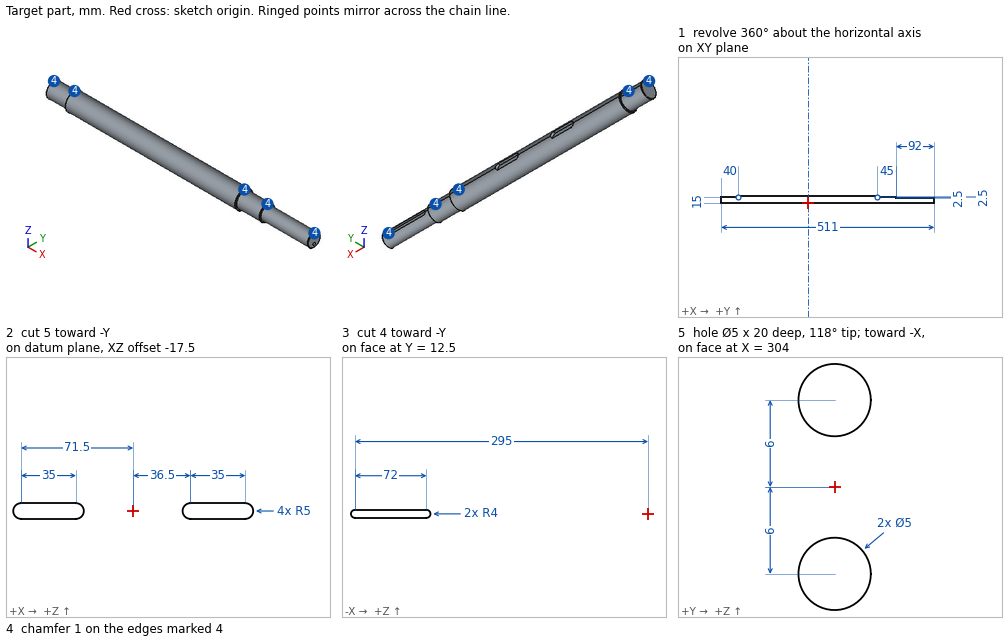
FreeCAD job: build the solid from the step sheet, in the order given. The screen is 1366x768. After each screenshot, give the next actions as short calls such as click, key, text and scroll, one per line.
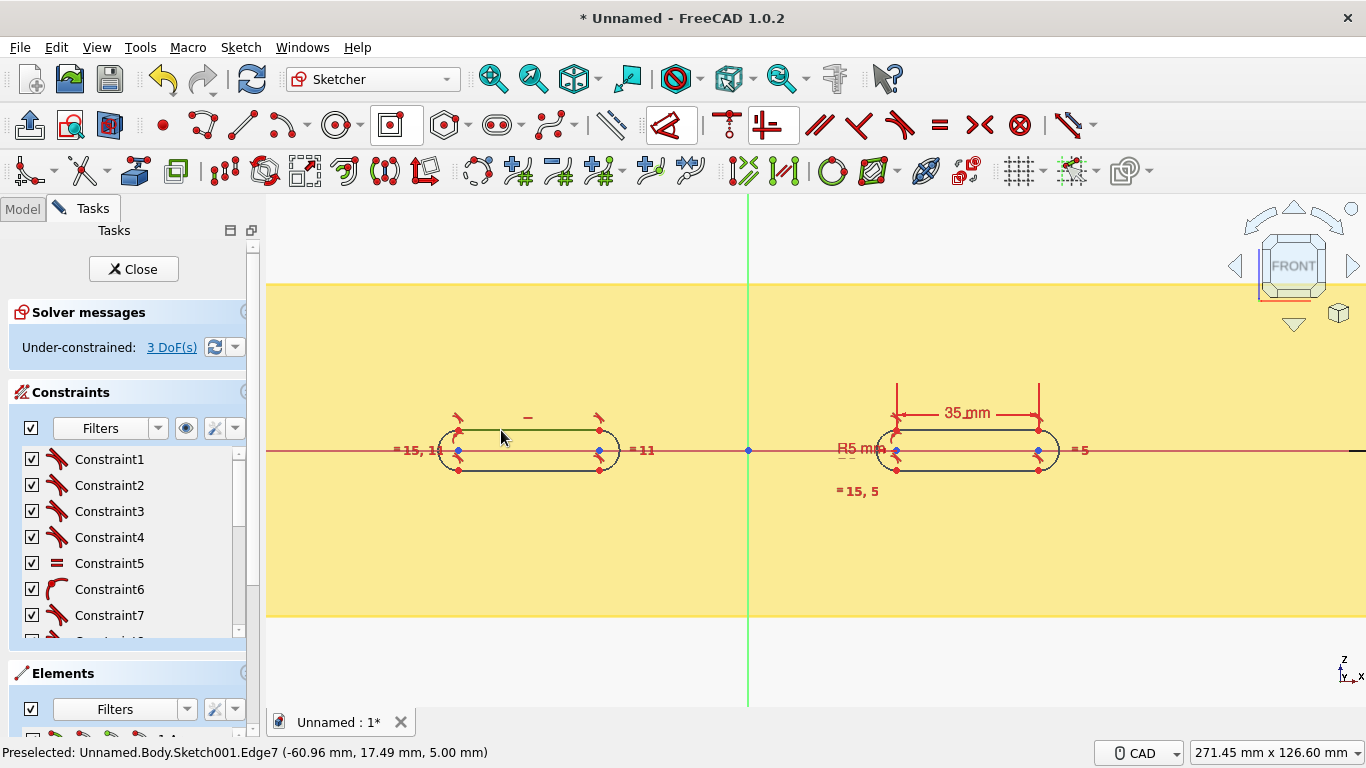
key(l)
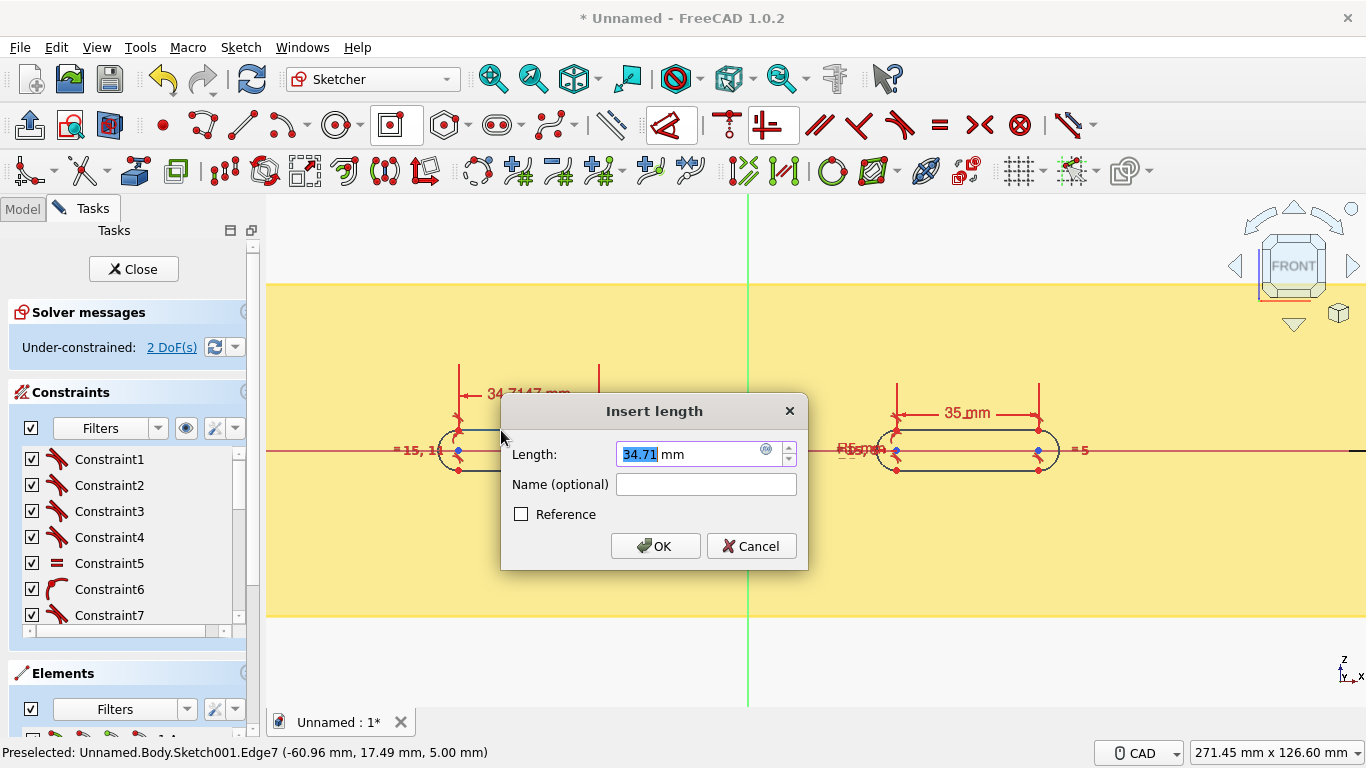
text(35)
key(Return)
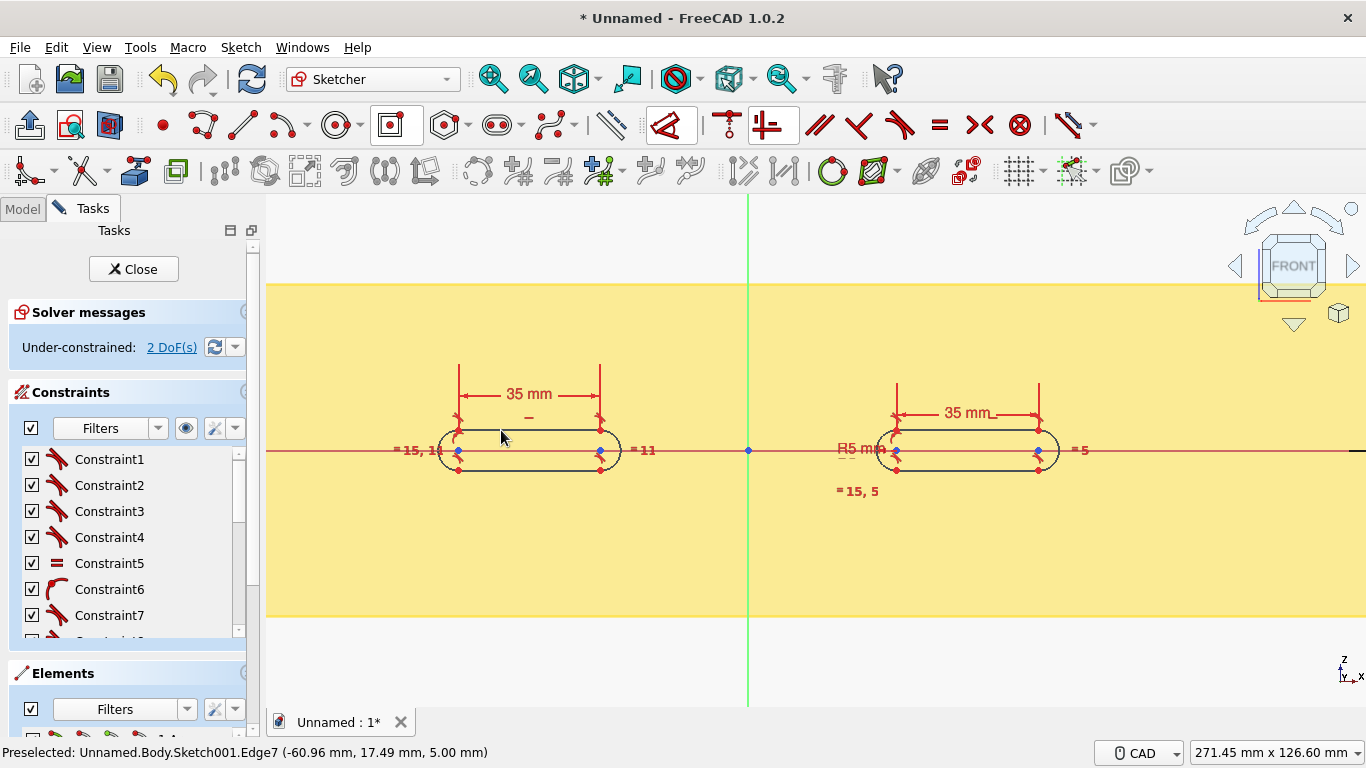
click(897, 430)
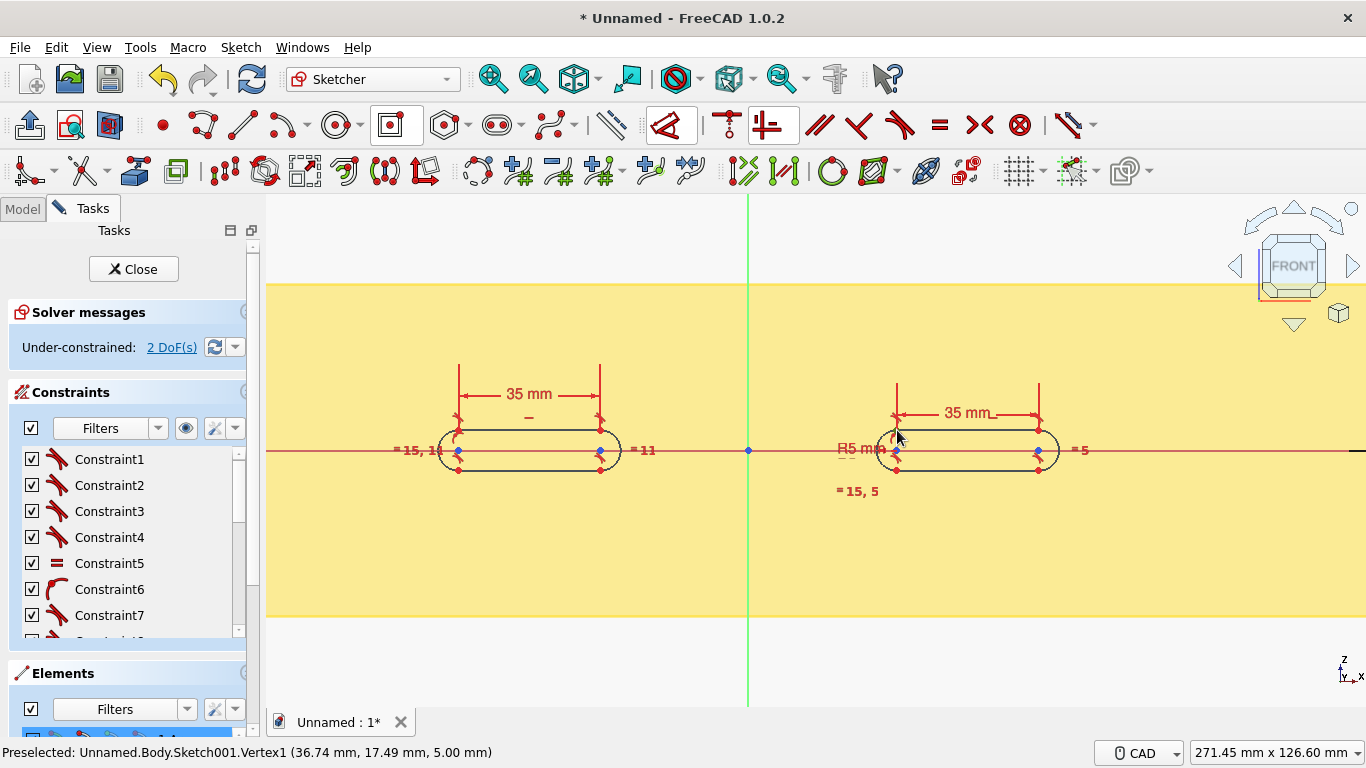
key(l)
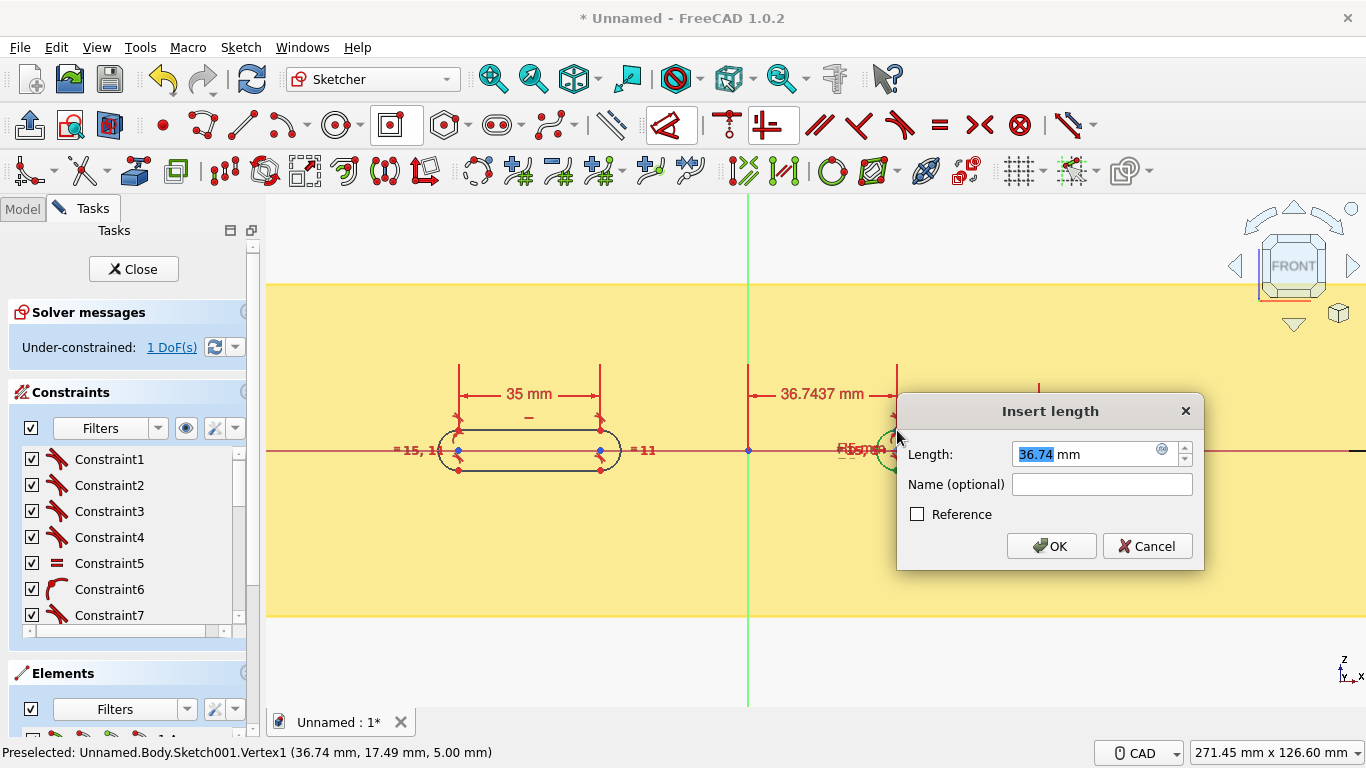
text(36.5)
key(Return)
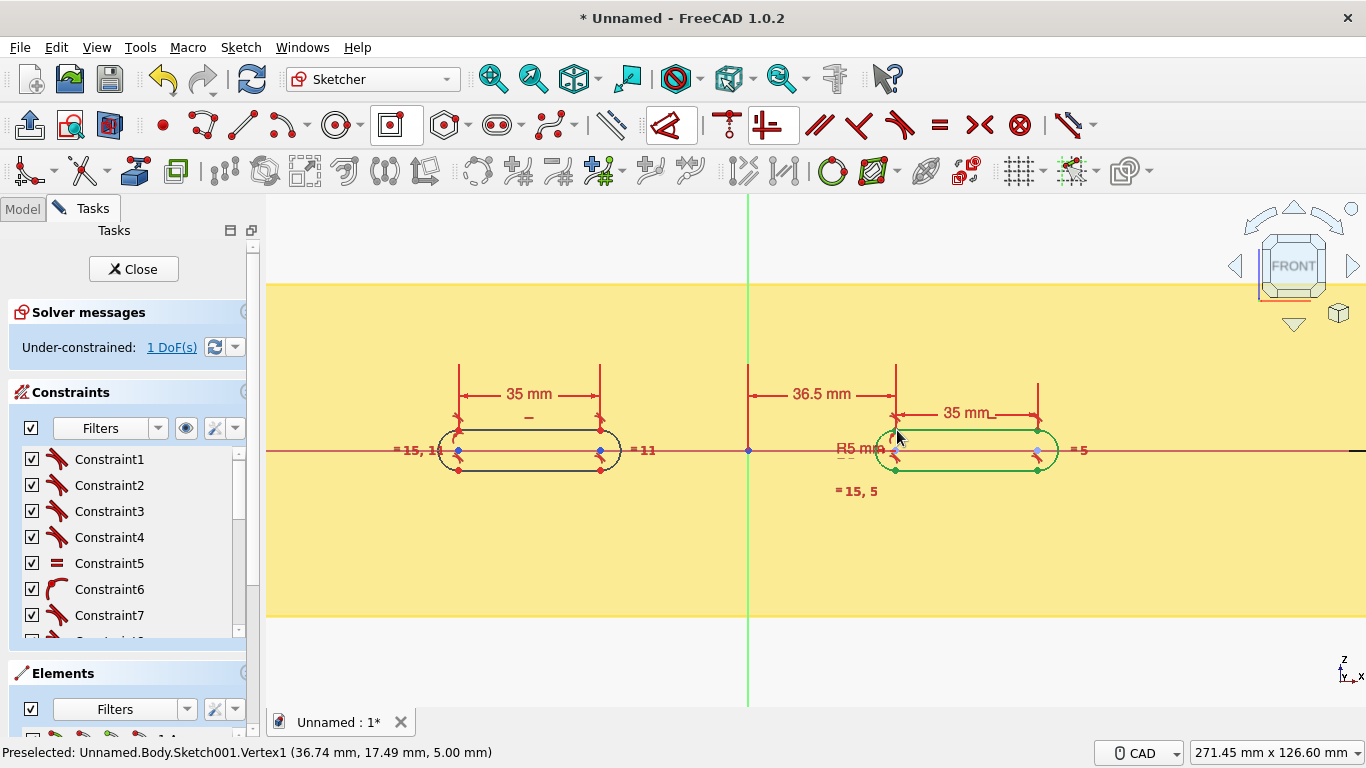
click(459, 430)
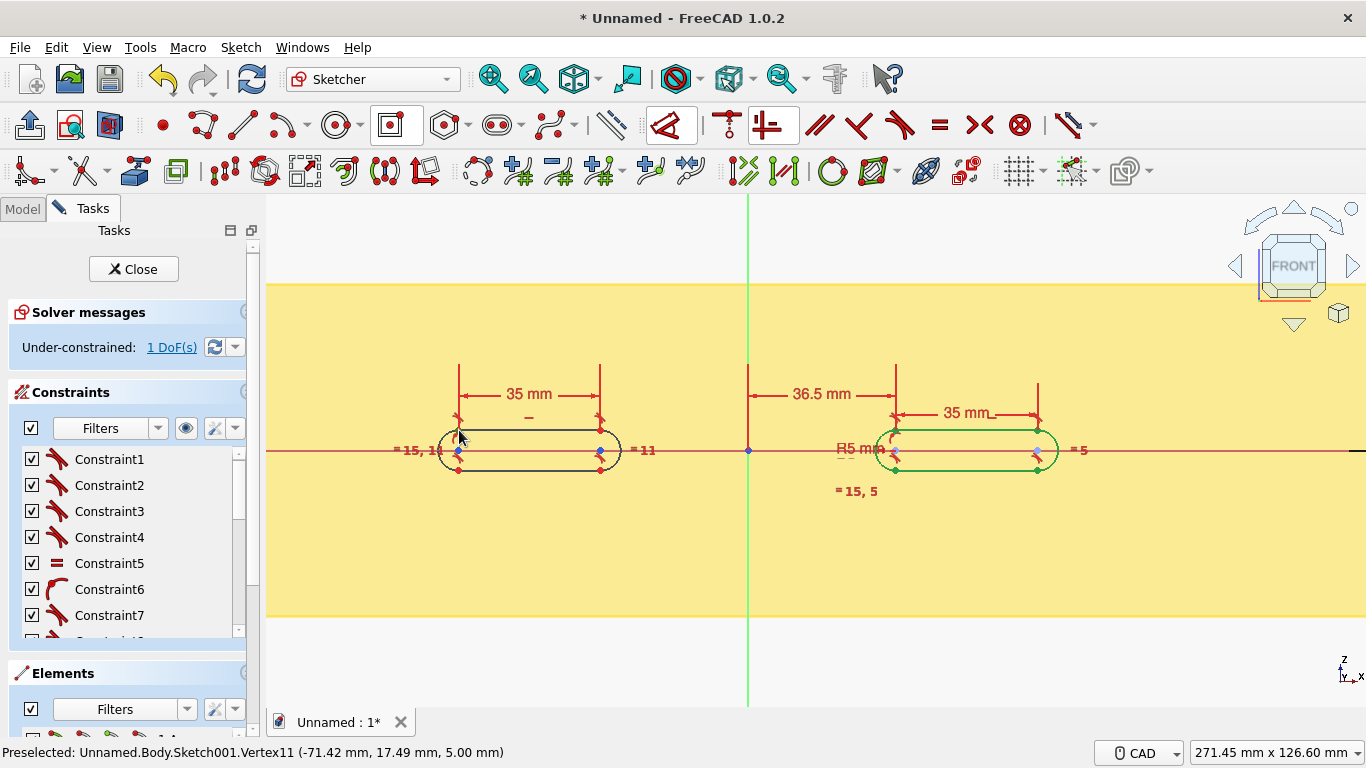
key(l)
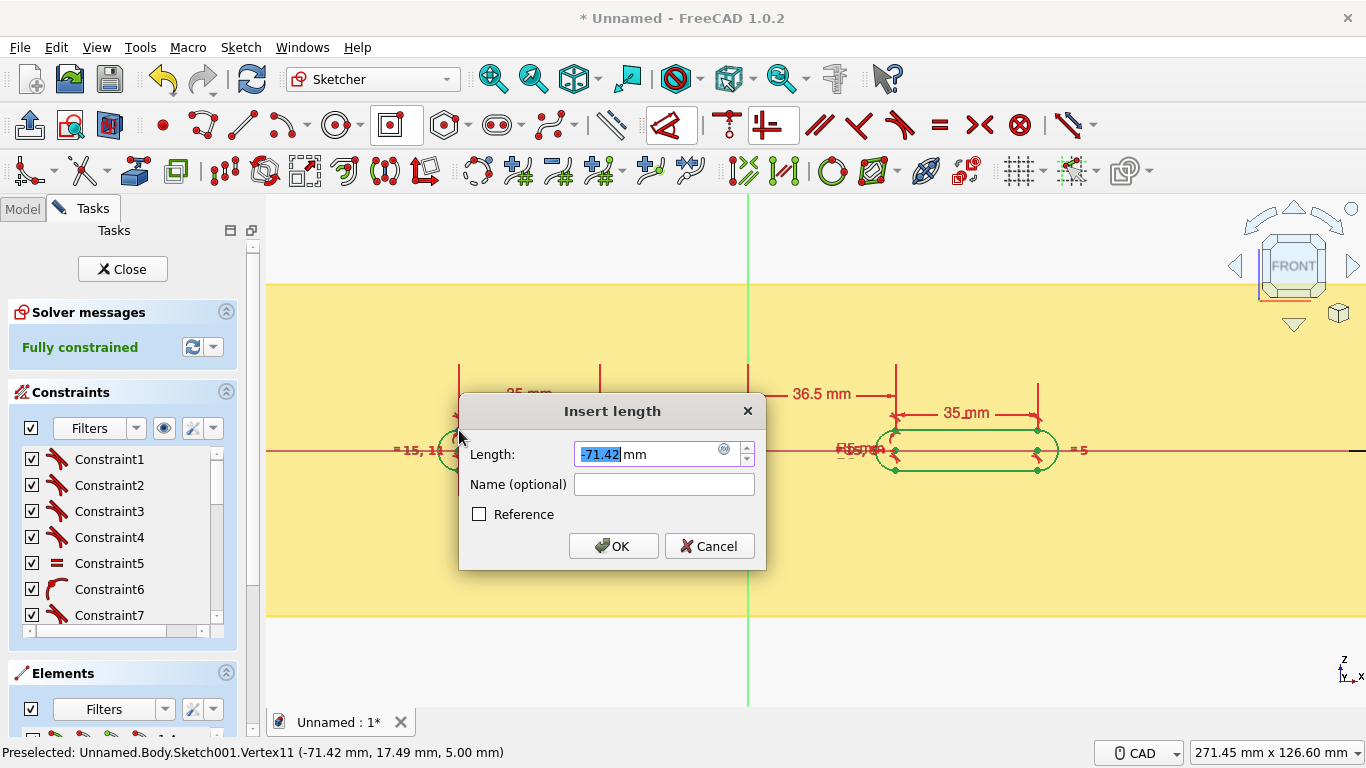
text(-71.5)
key(Return)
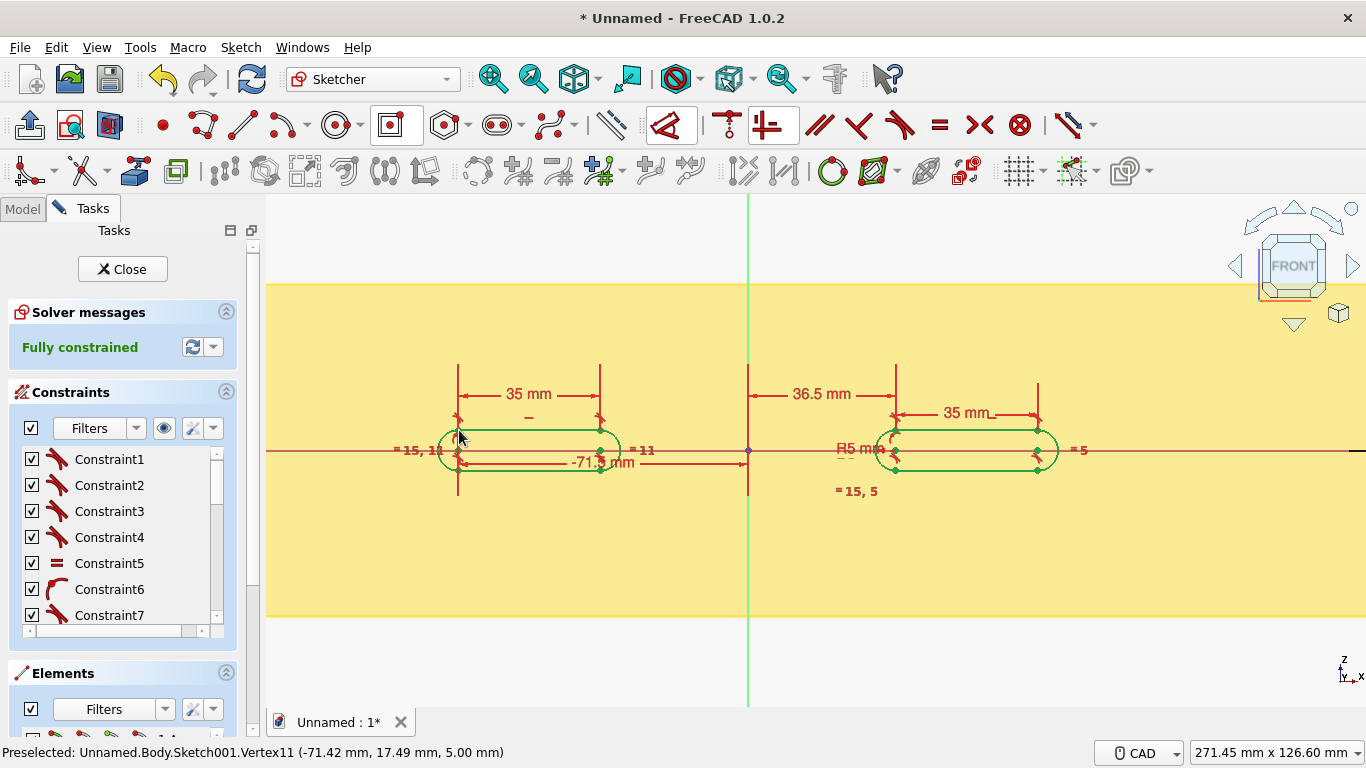
click(123, 269)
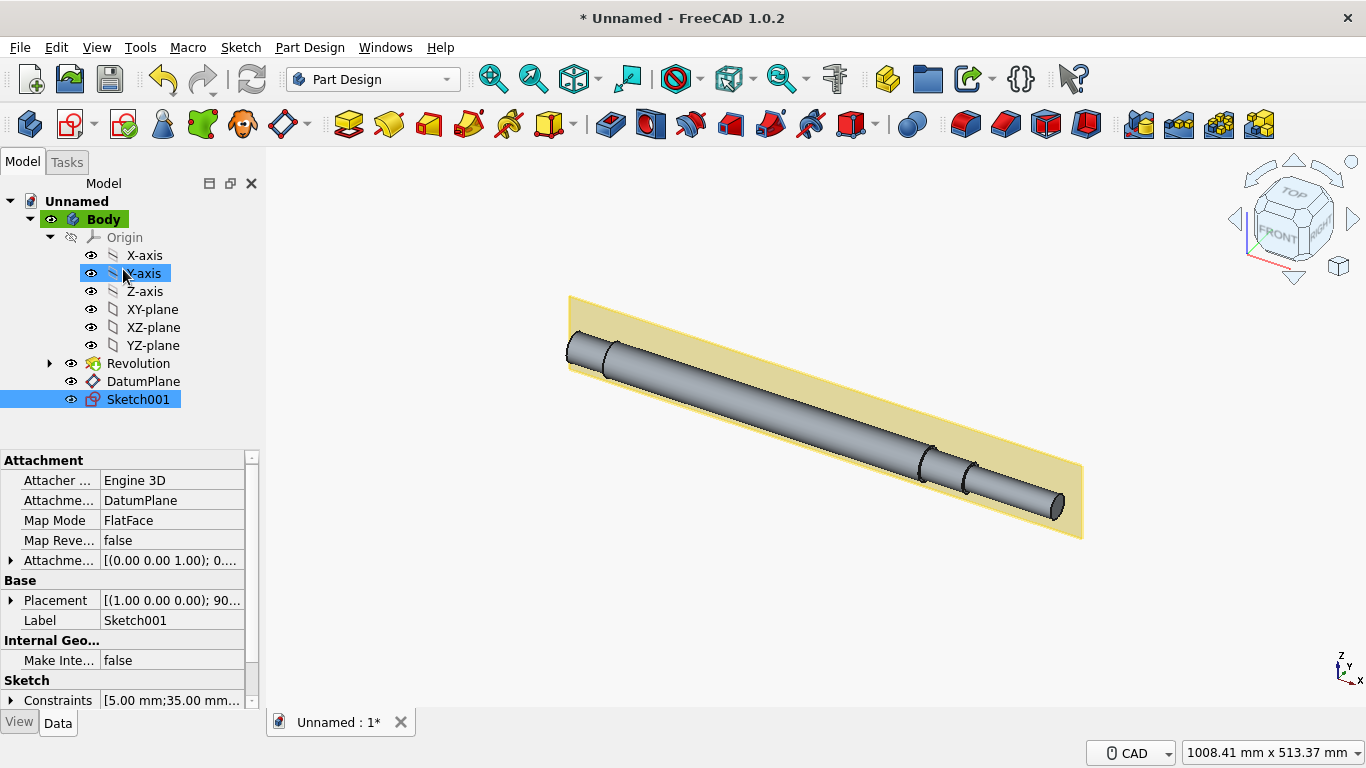
click(612, 124)